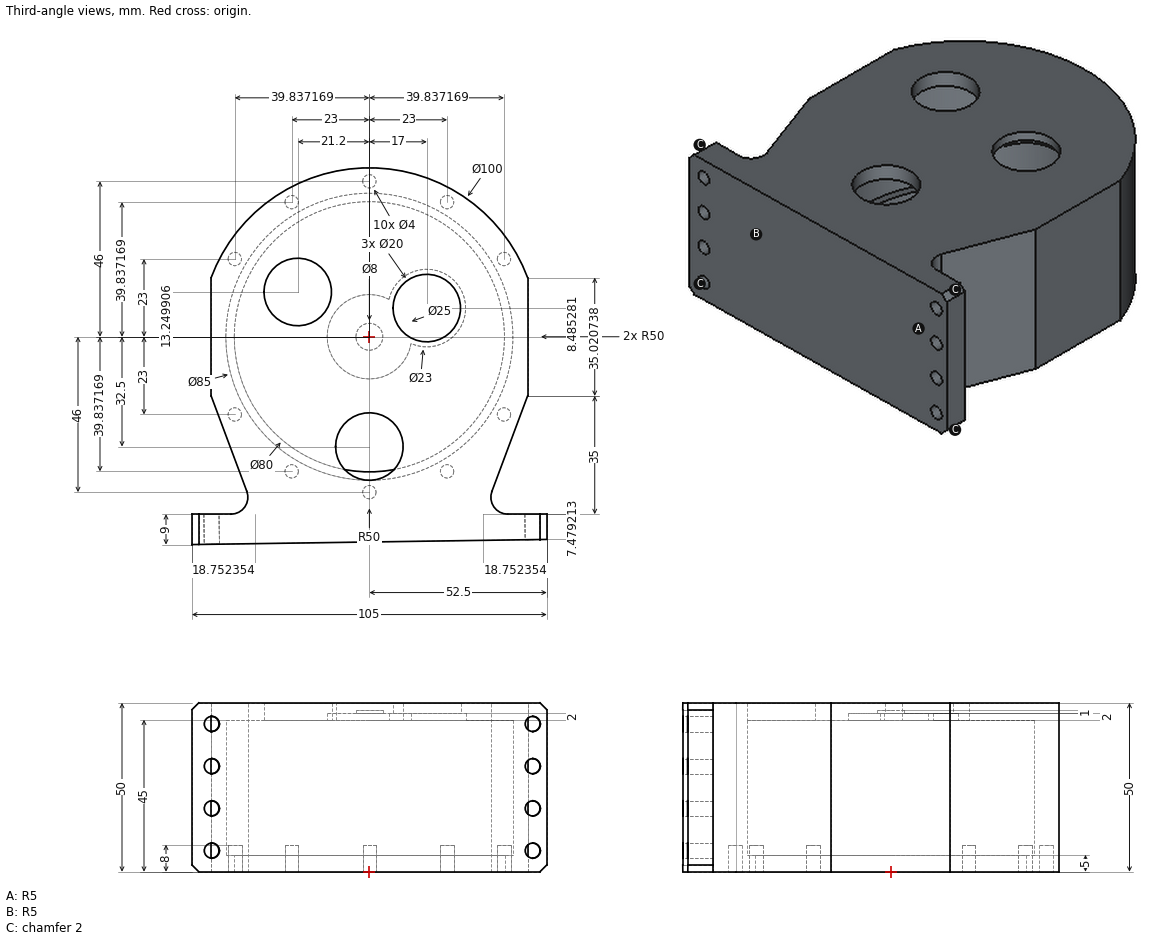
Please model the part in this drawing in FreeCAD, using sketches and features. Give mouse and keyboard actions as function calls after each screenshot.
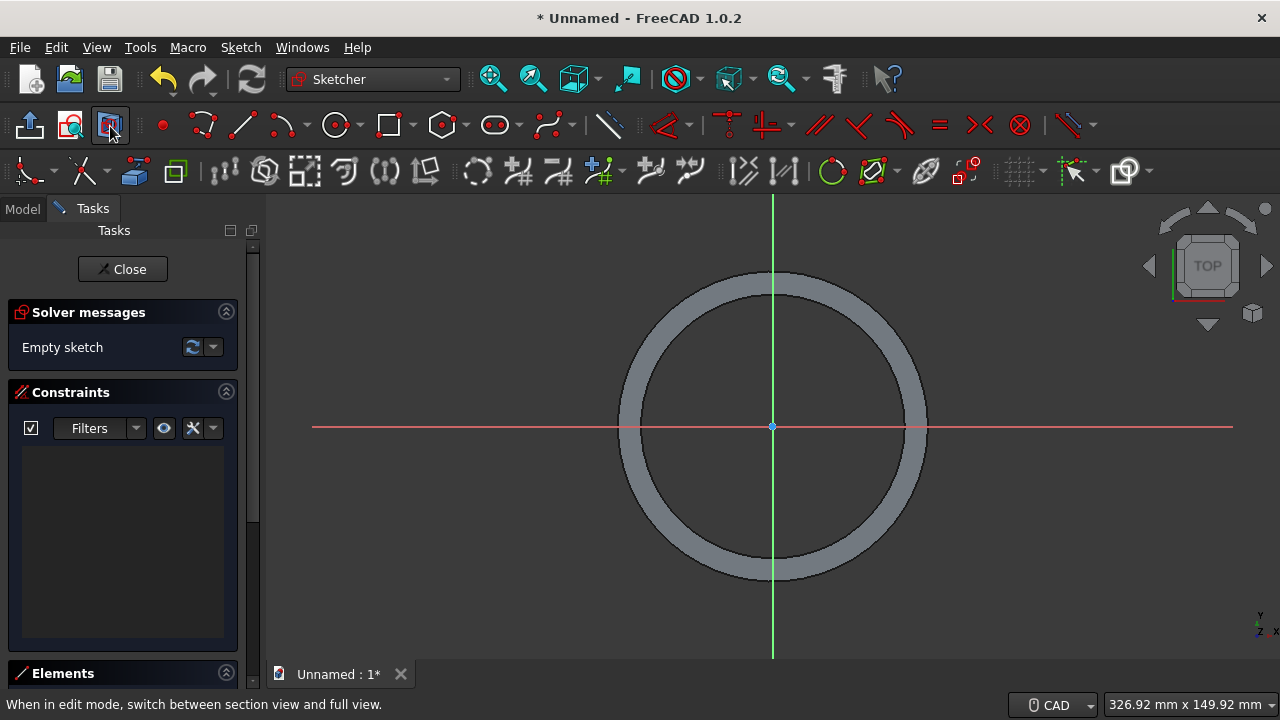
scroll(396, 222, down, 1)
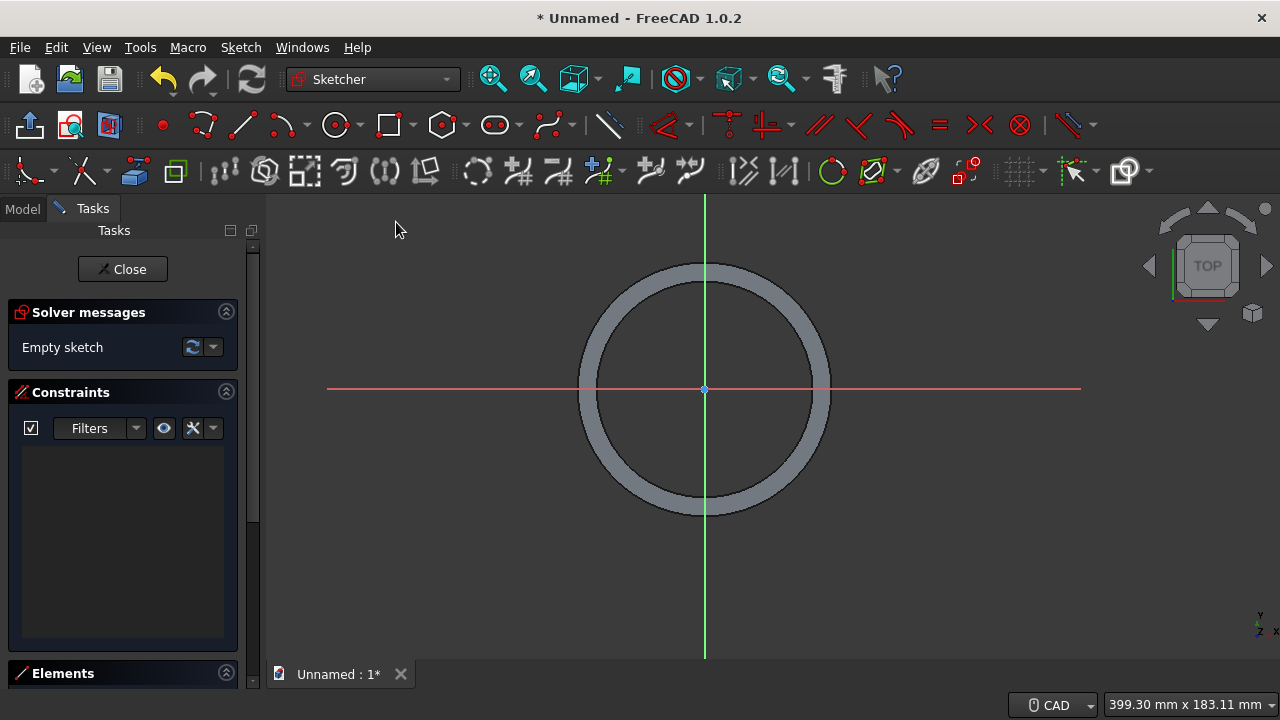
scroll(705, 517, up, 3)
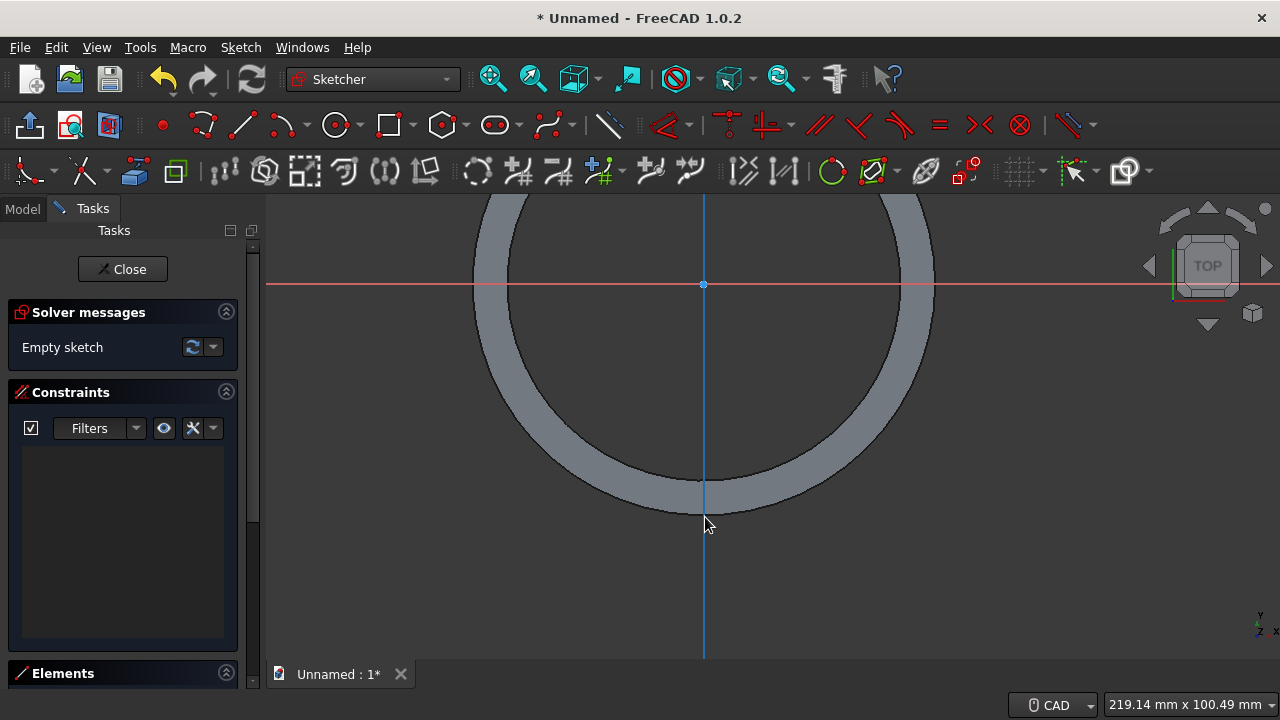
key(g)
key(m)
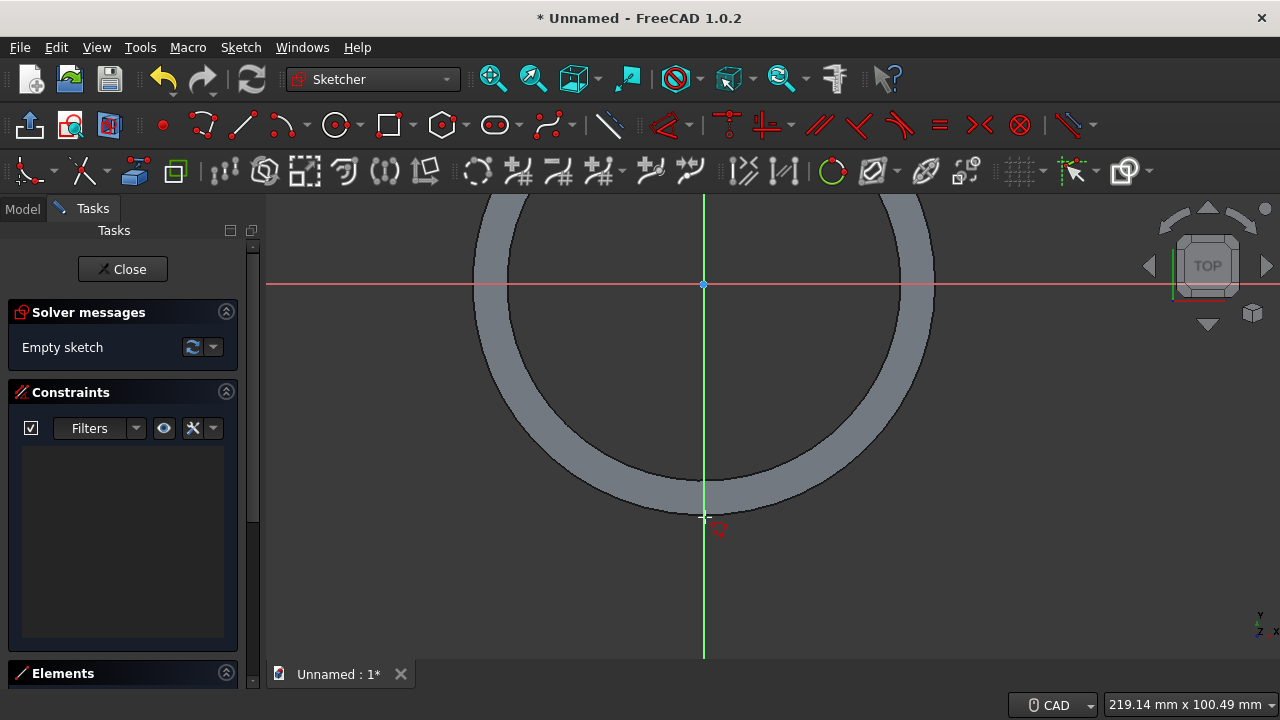
click(921, 365)
click(860, 527)
click(947, 527)
click(947, 562)
click(461, 585)
click(461, 527)
click(548, 527)
click(487, 365)
right_click(487, 365)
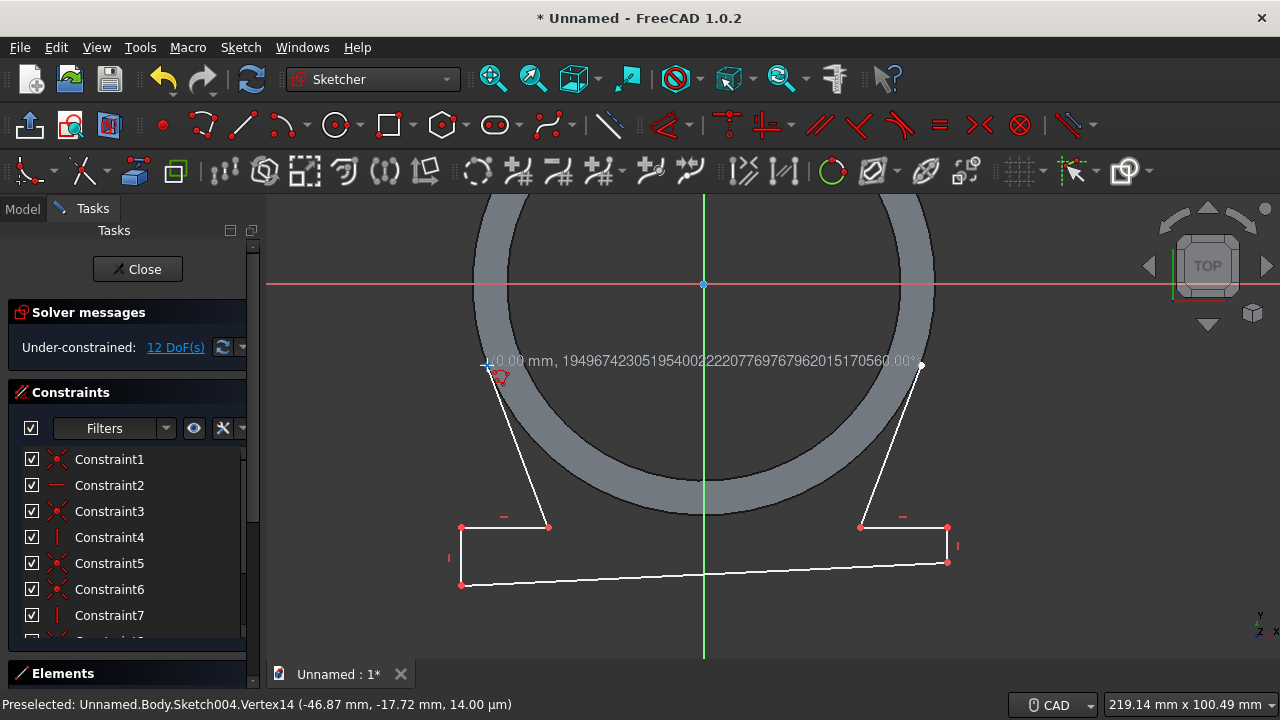
click(310, 126)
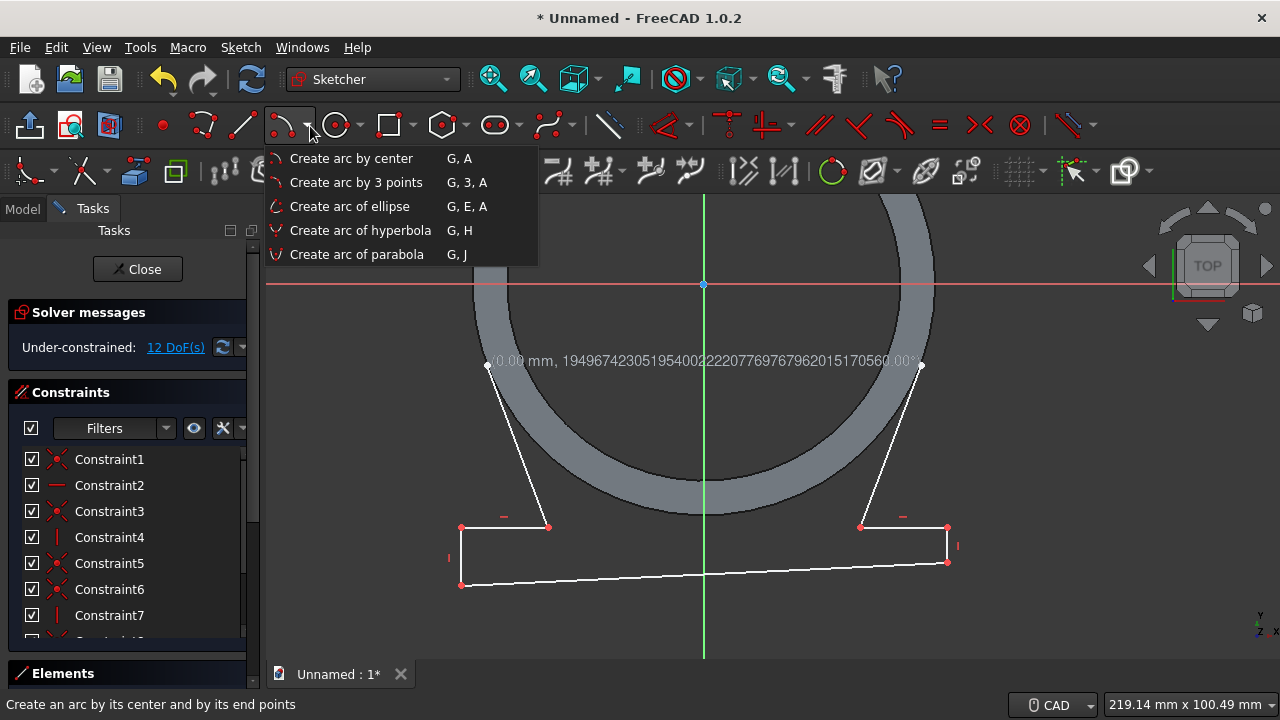
click(402, 182)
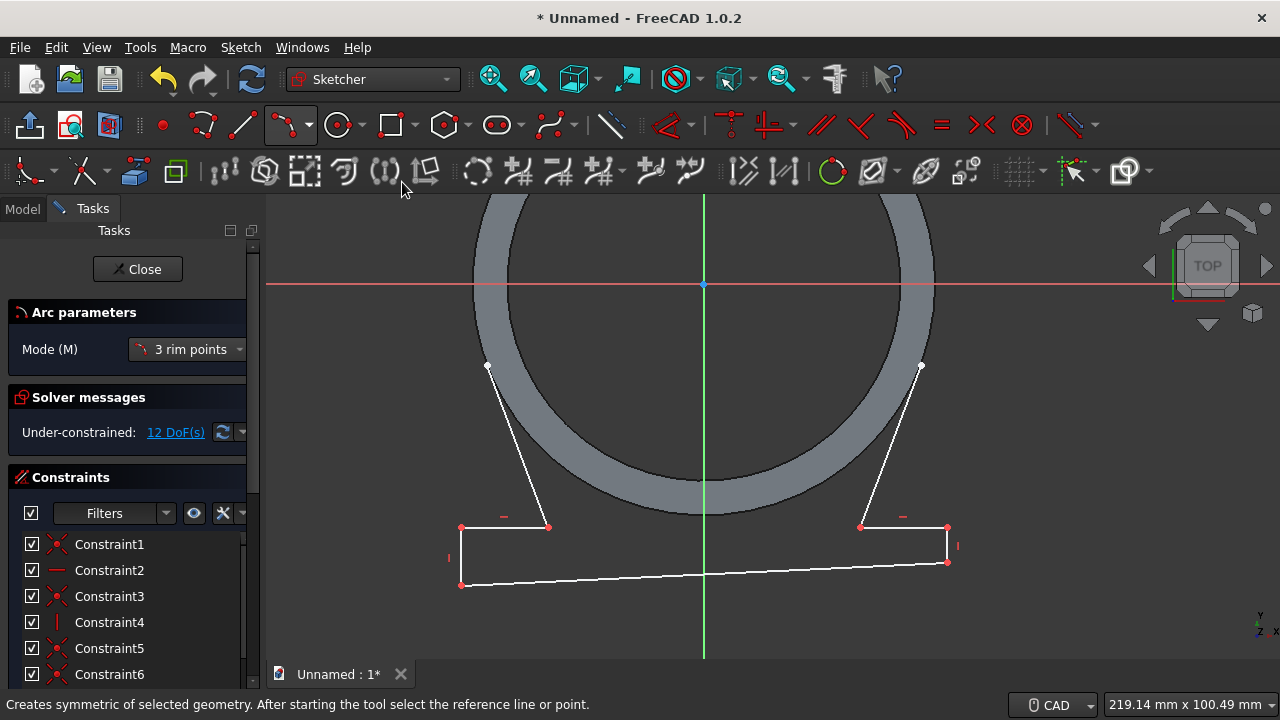
click(487, 366)
click(921, 366)
click(648, 509)
key(Escape)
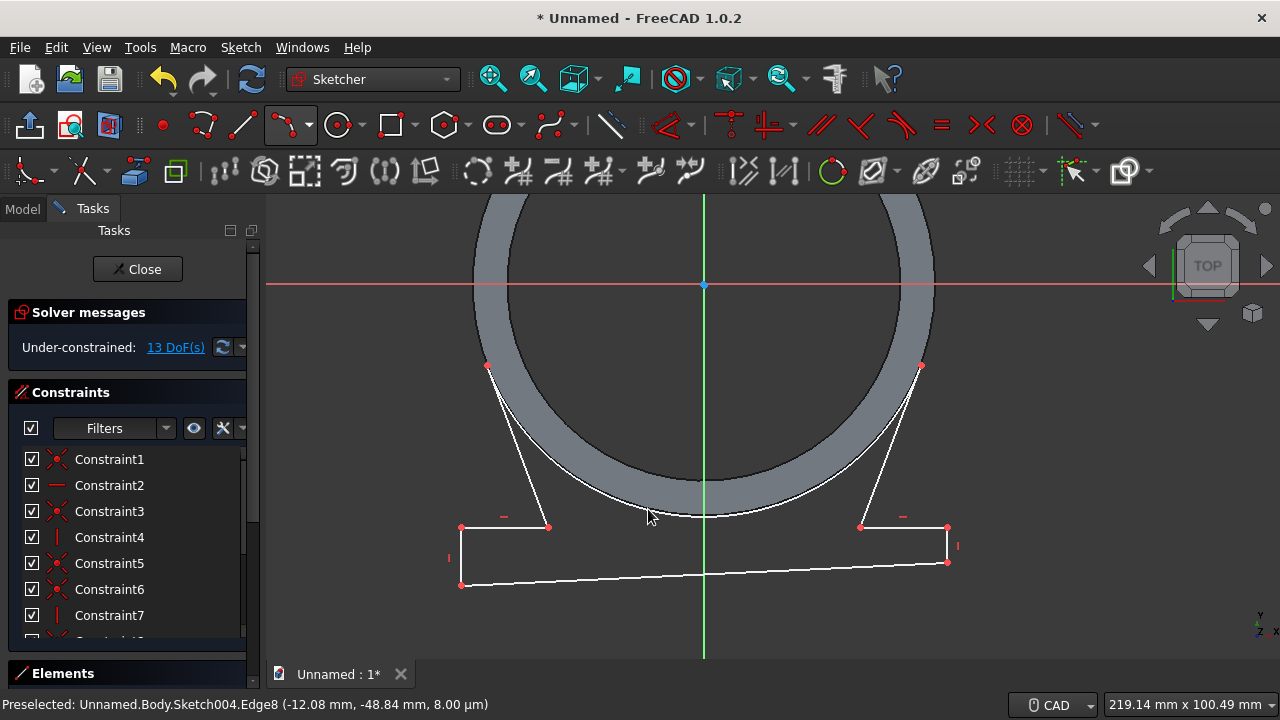
click(878, 479)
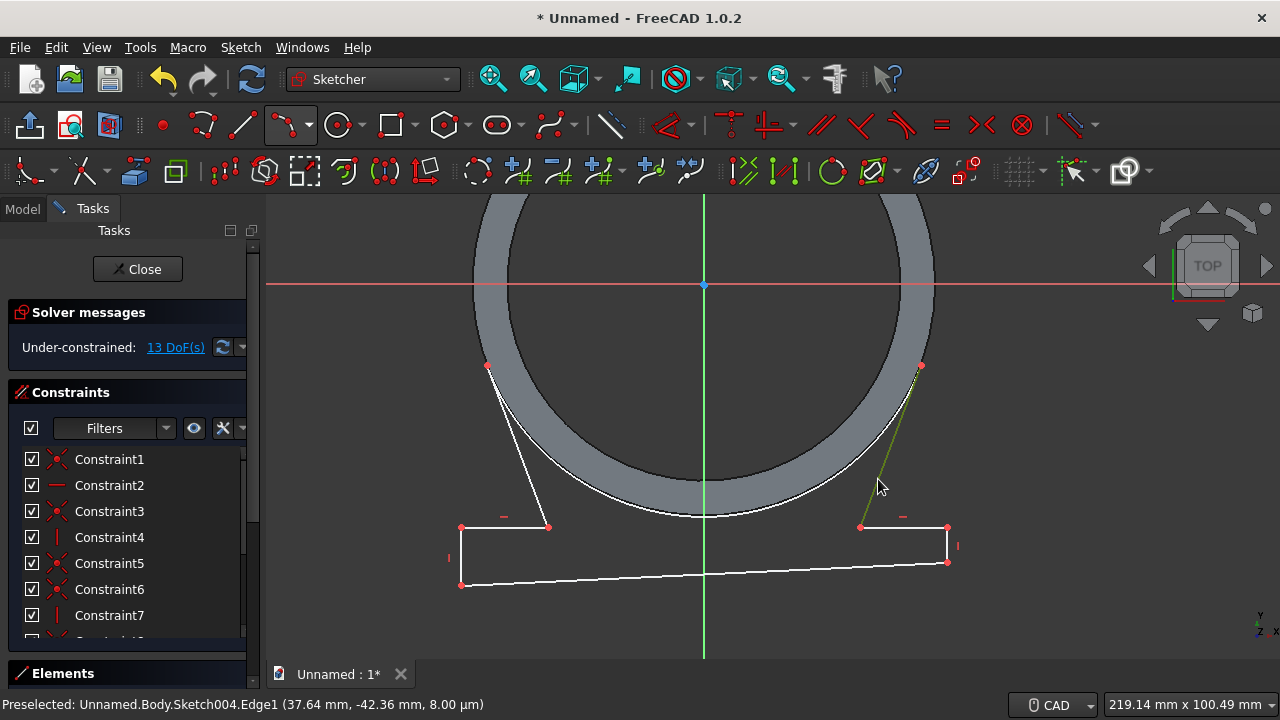
click(596, 490)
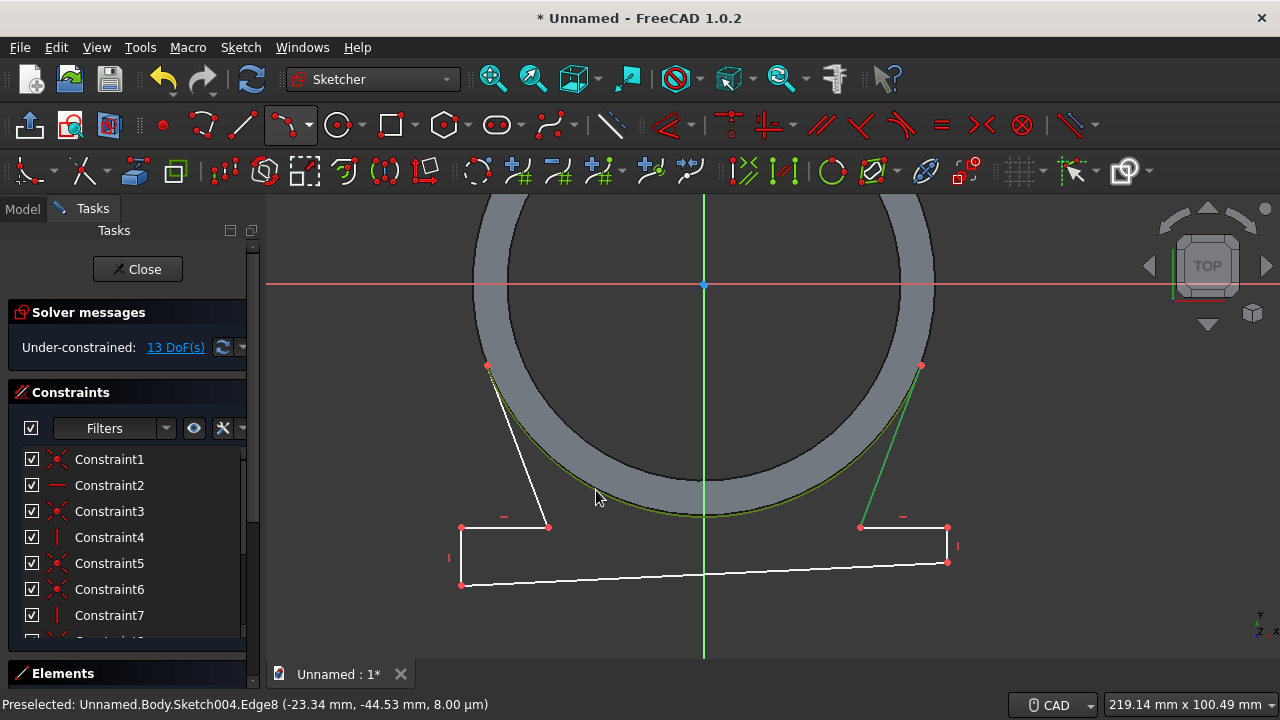
key(t)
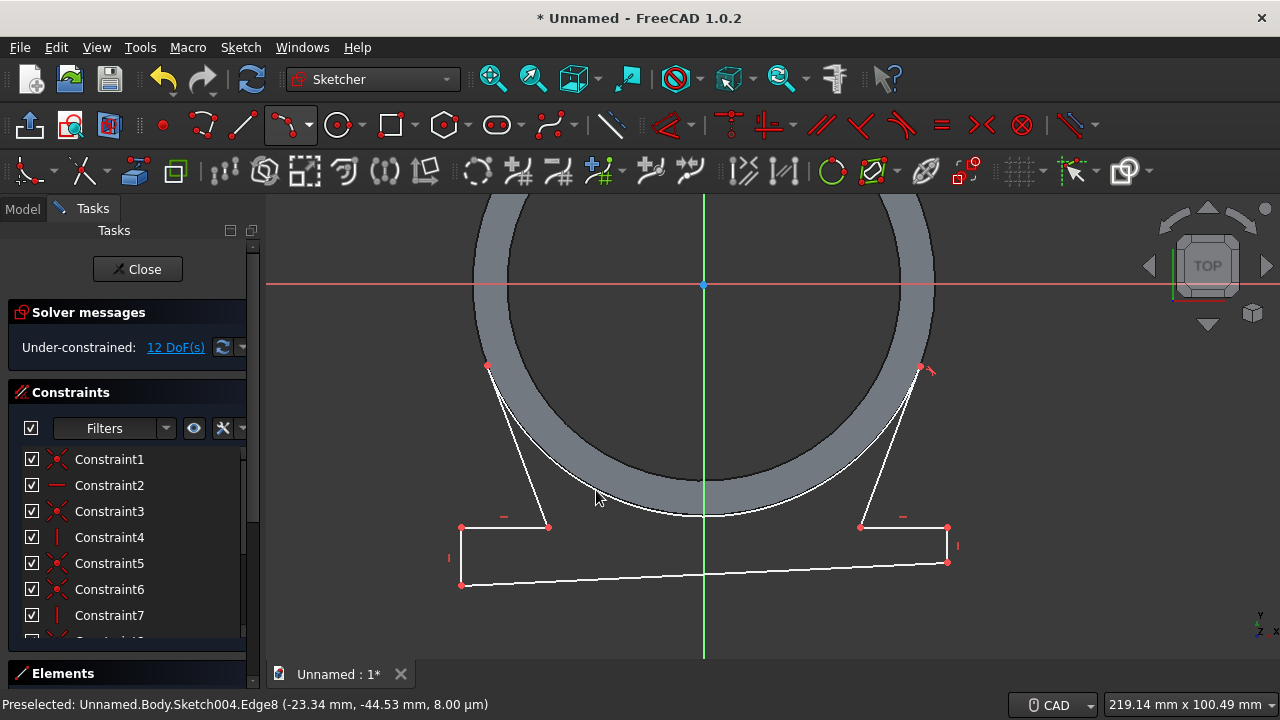
click(530, 479)